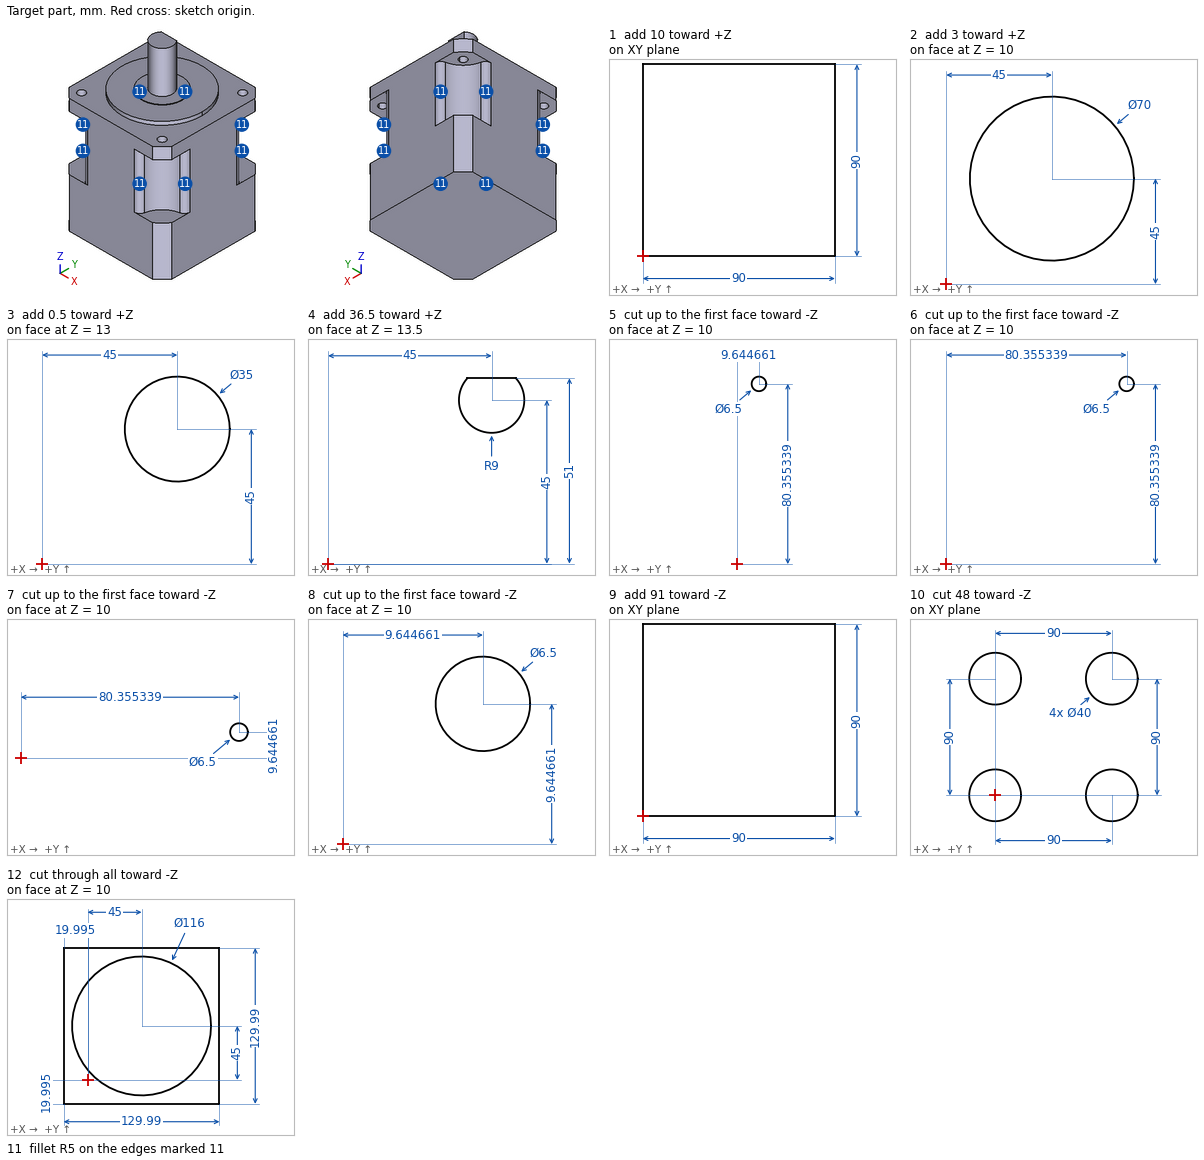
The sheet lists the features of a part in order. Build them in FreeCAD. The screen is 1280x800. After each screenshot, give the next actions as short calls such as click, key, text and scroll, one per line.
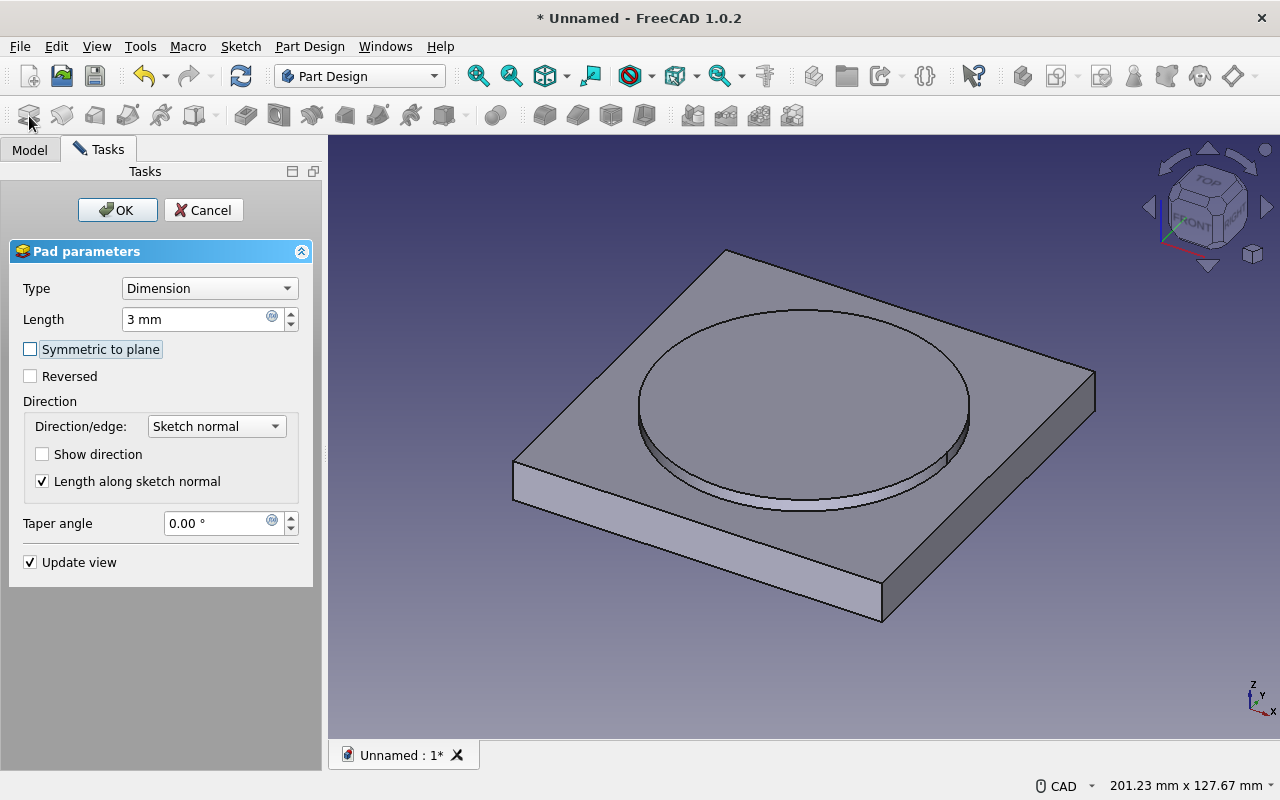
click(118, 210)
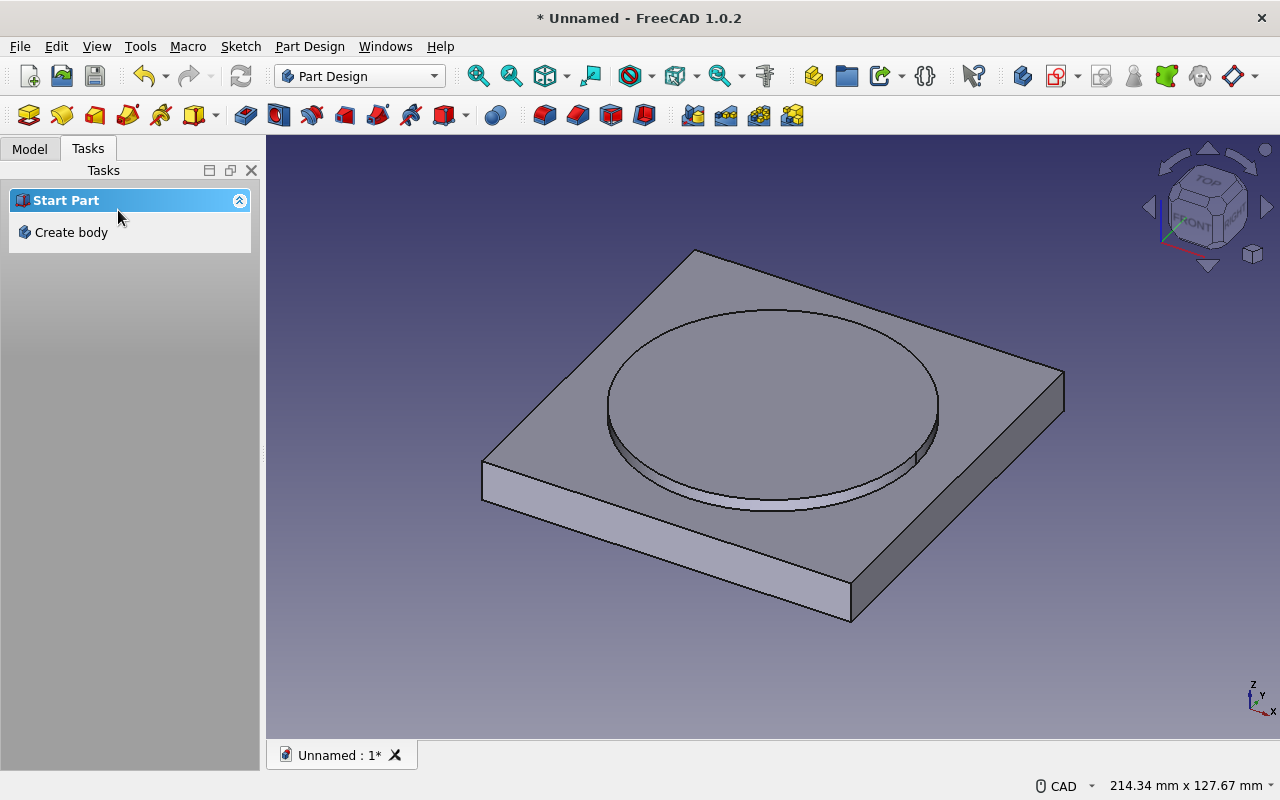
click(773, 404)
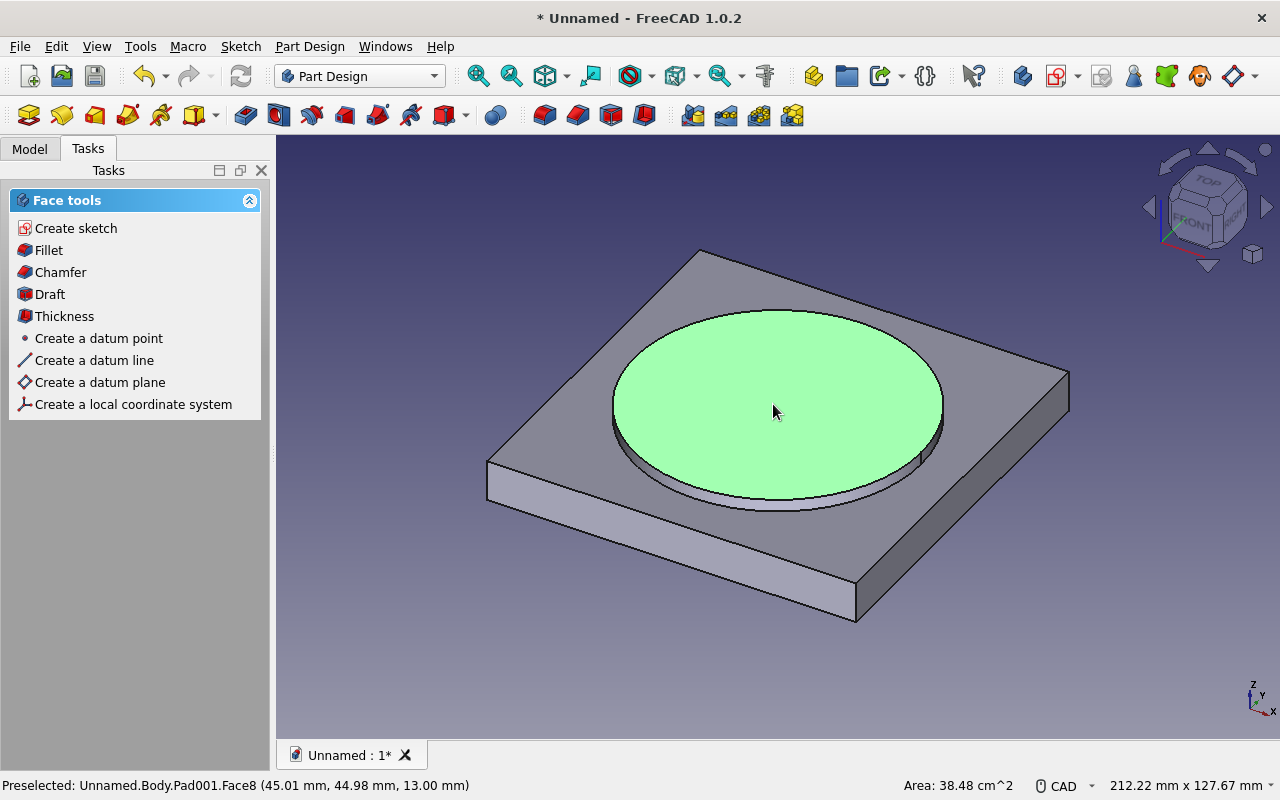
click(1056, 76)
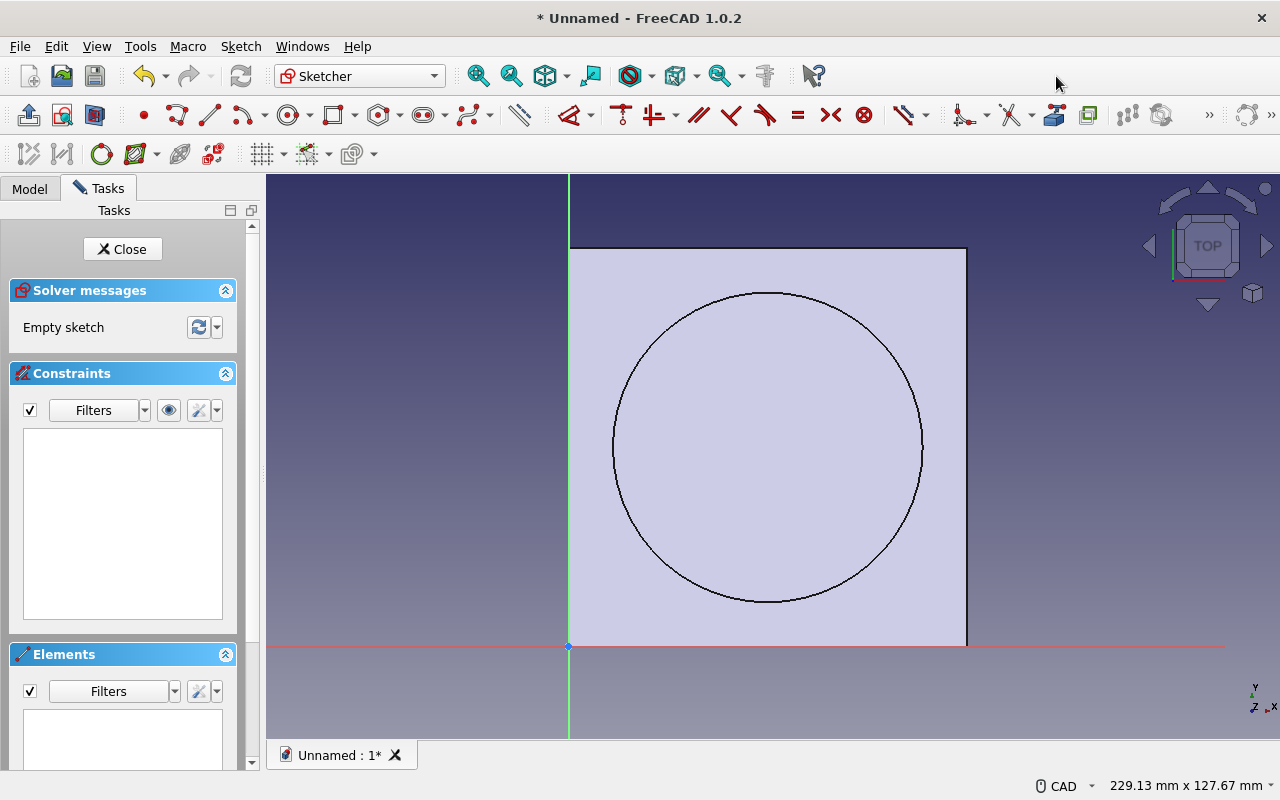
key(g)
key(c)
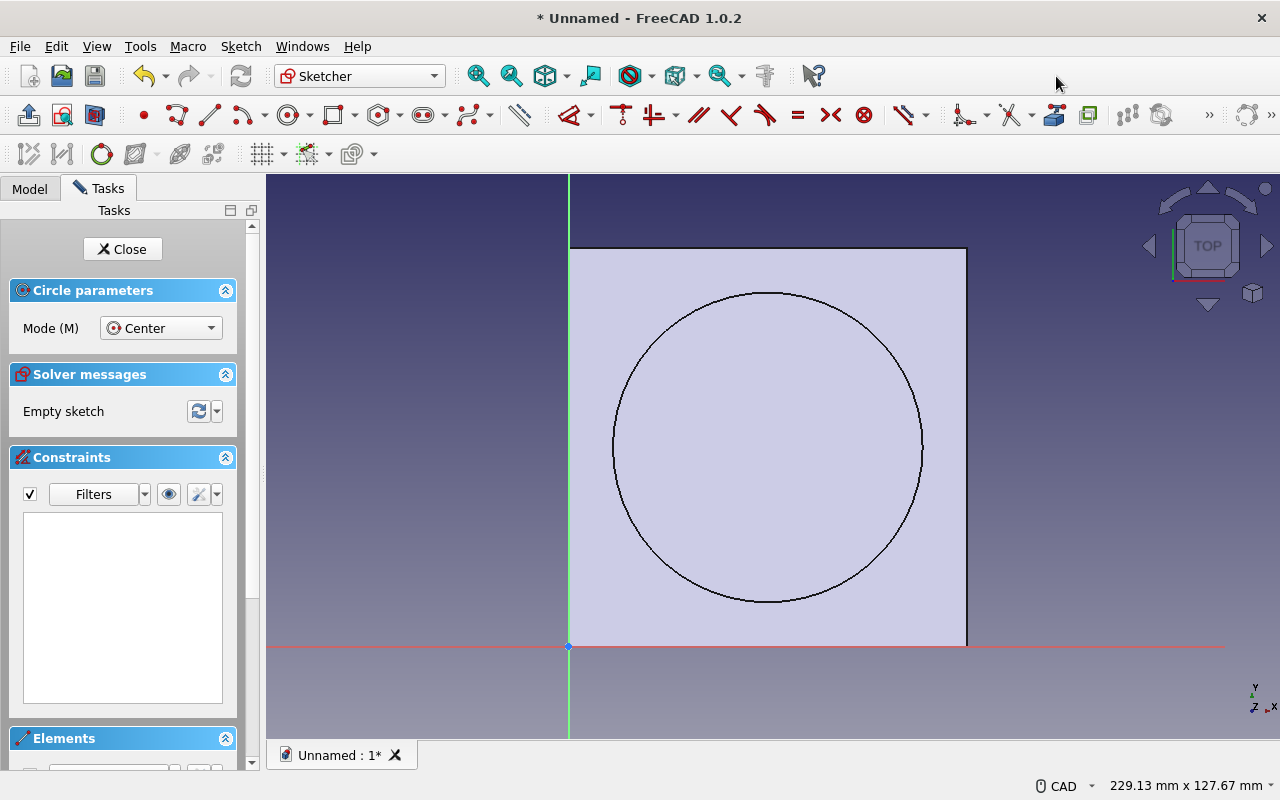
click(768, 447)
move(823, 393)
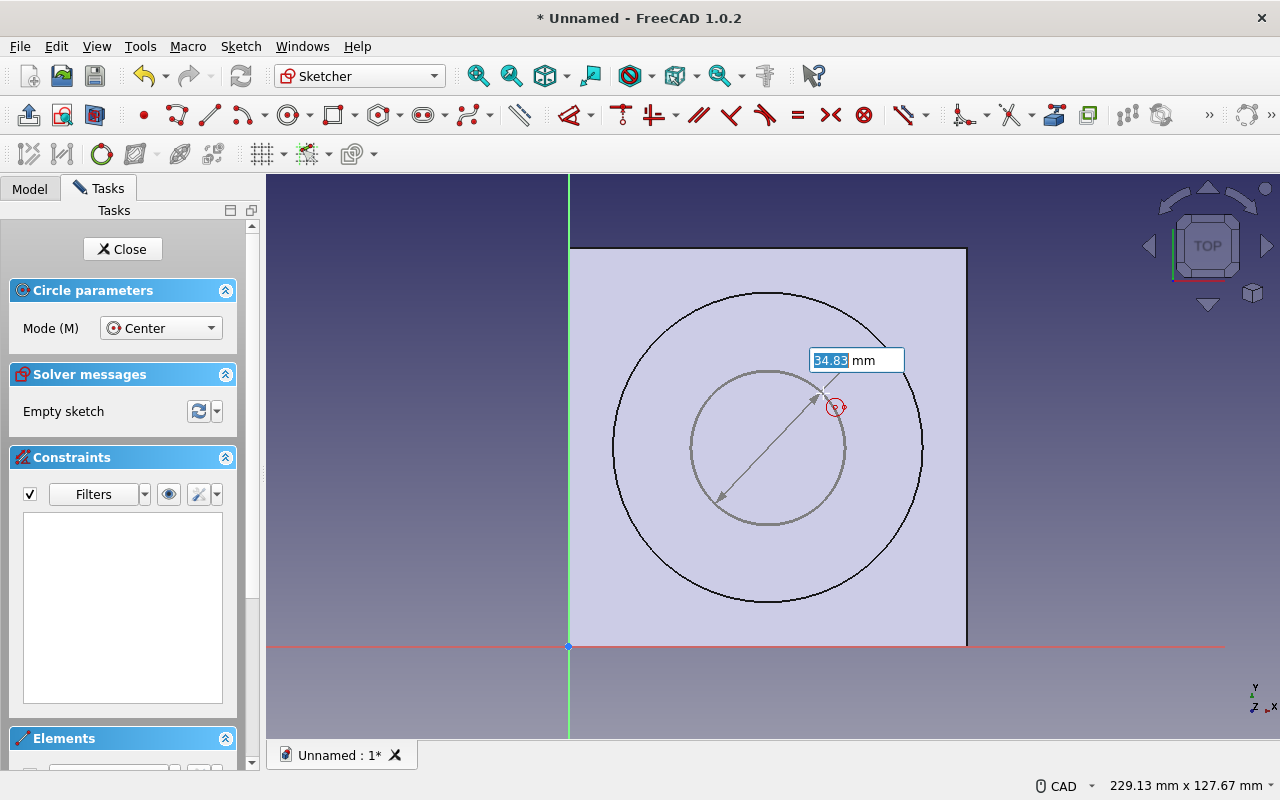
text(35)
key(Return)
key(Escape)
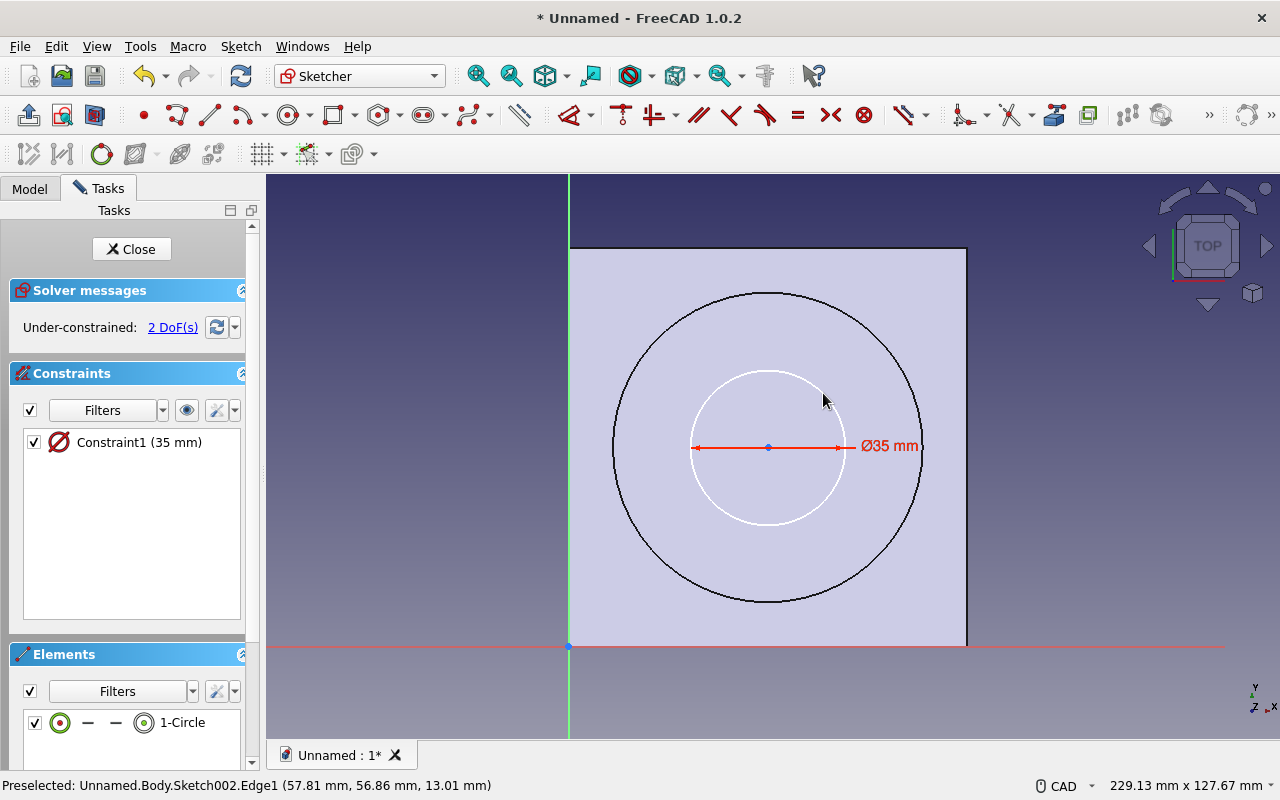
click(768, 448)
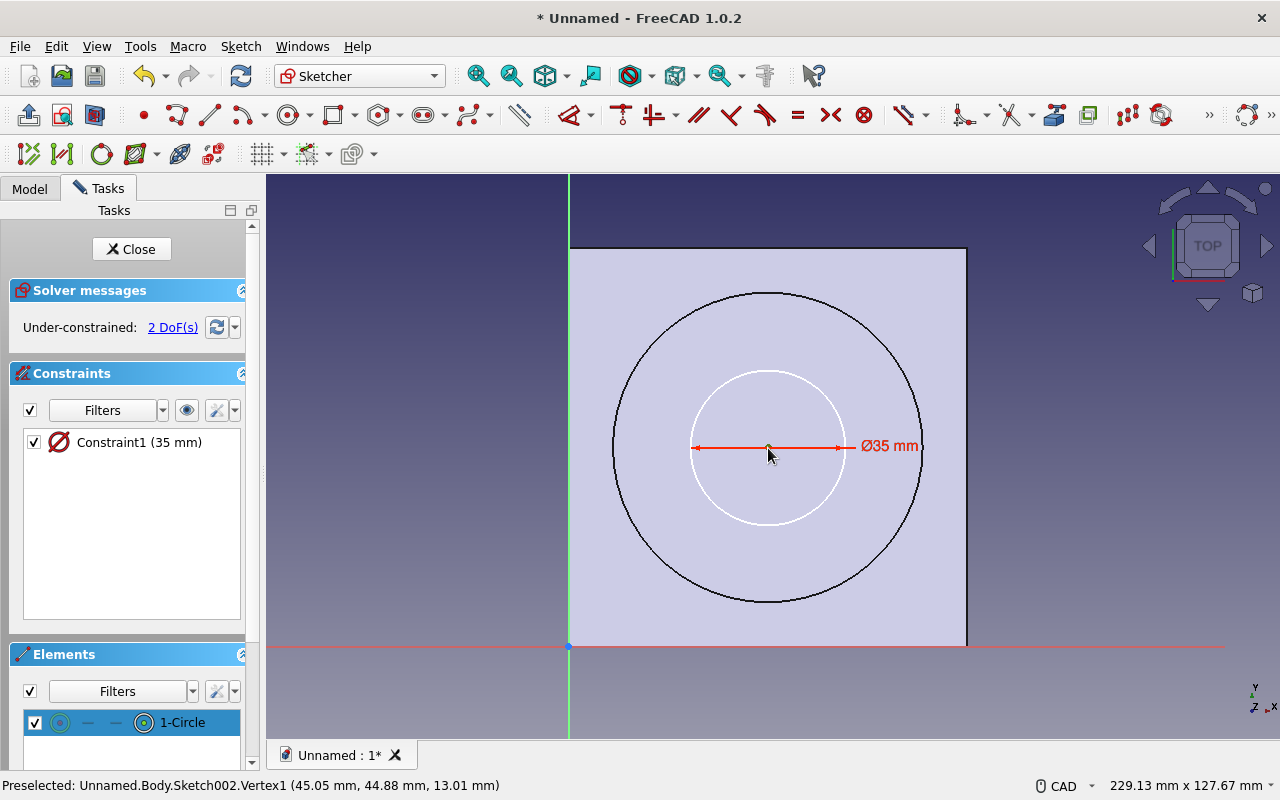
click(590, 116)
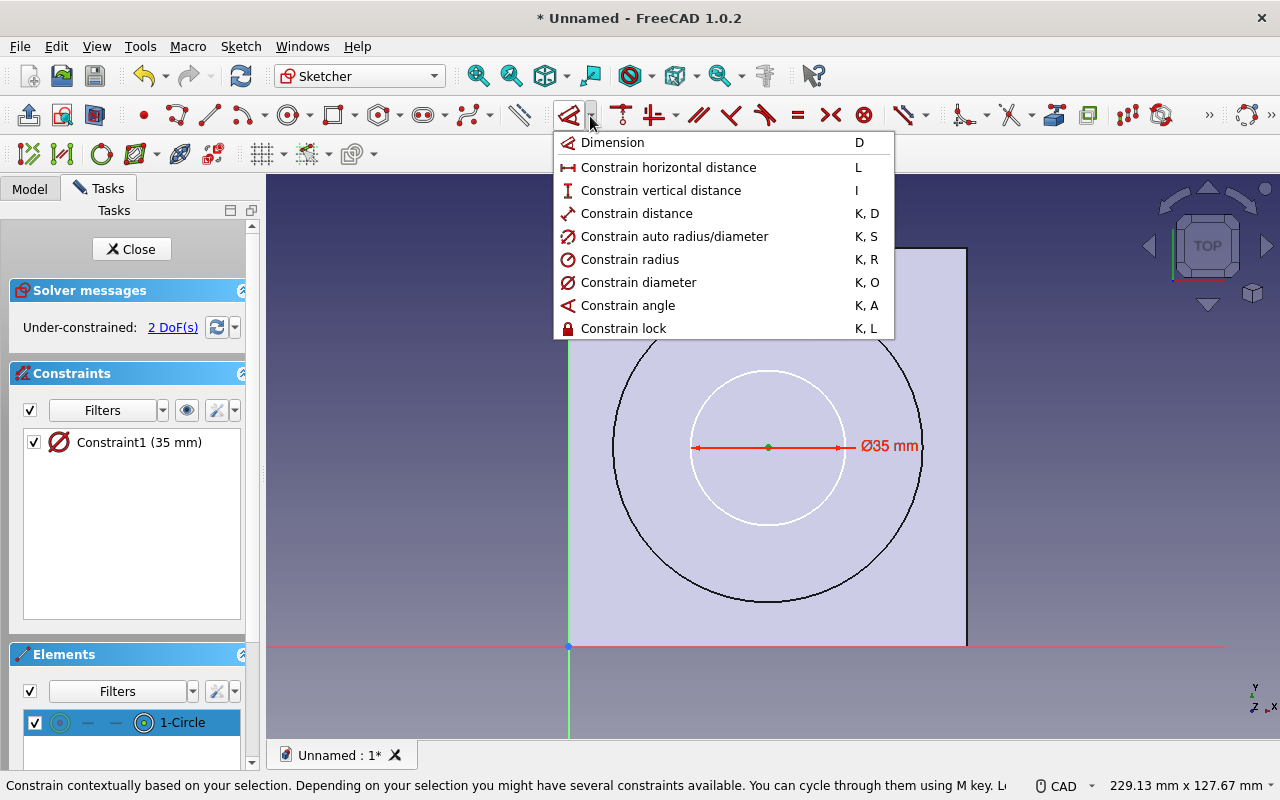
click(724, 168)